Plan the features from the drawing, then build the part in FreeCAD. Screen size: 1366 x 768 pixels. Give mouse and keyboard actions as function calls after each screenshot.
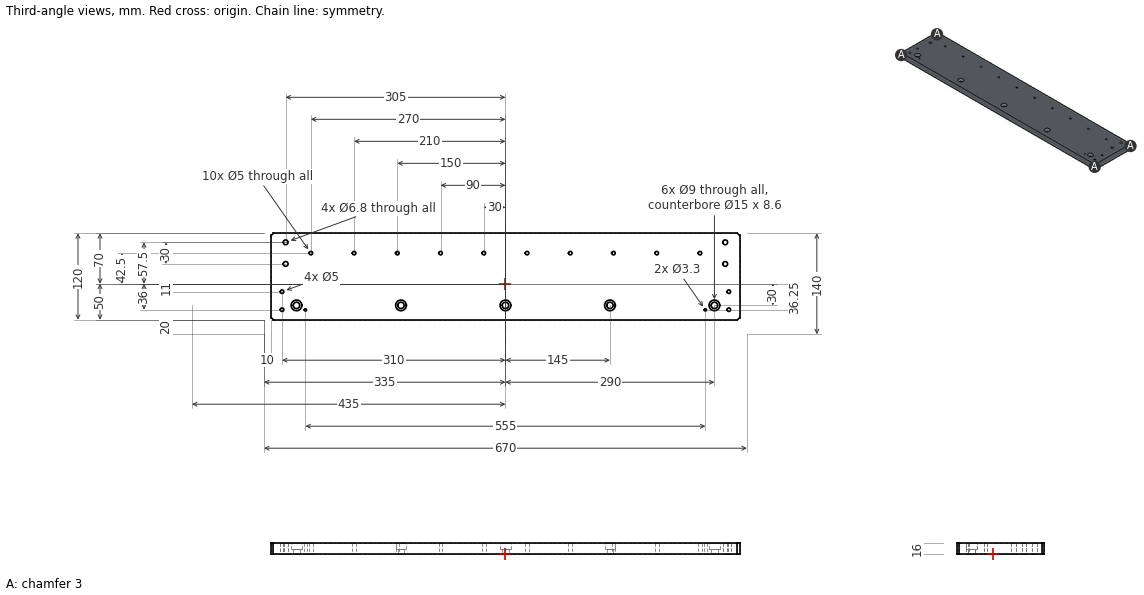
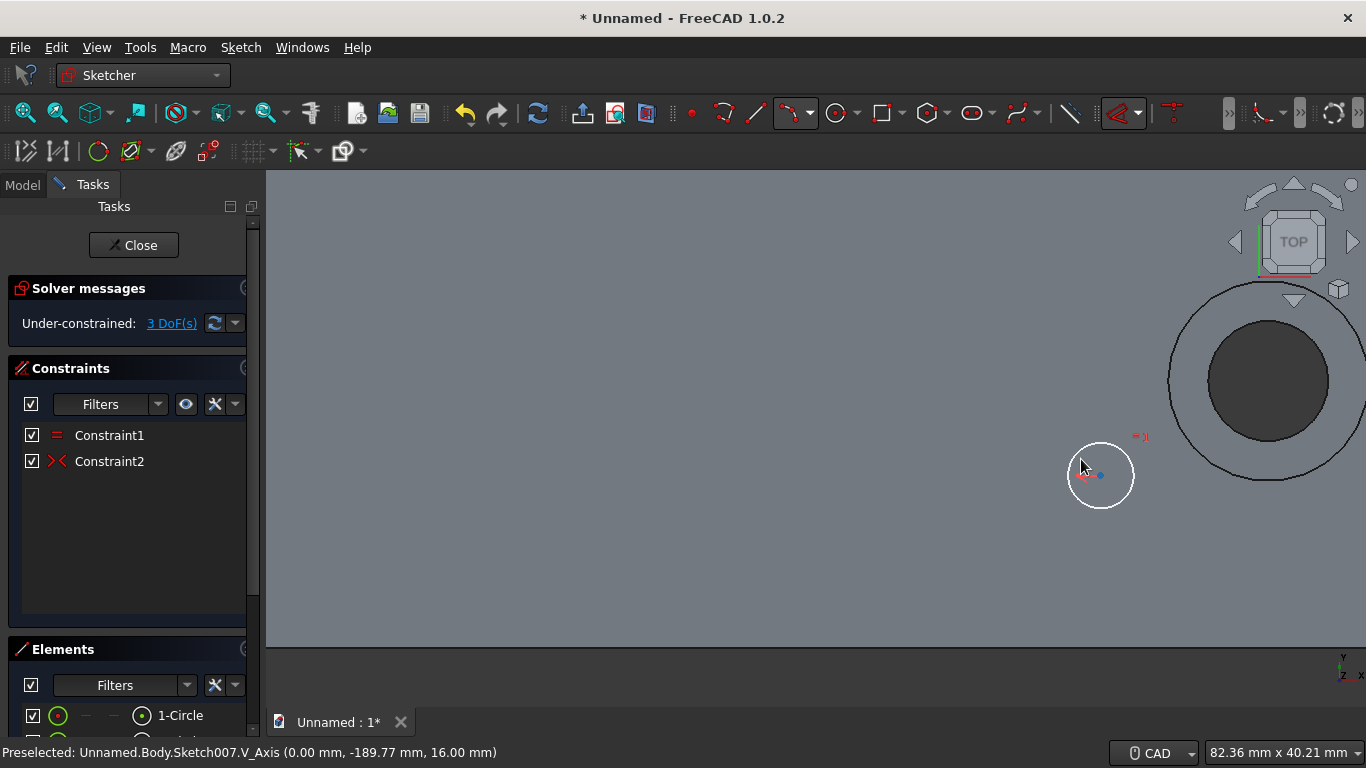
click(1078, 453)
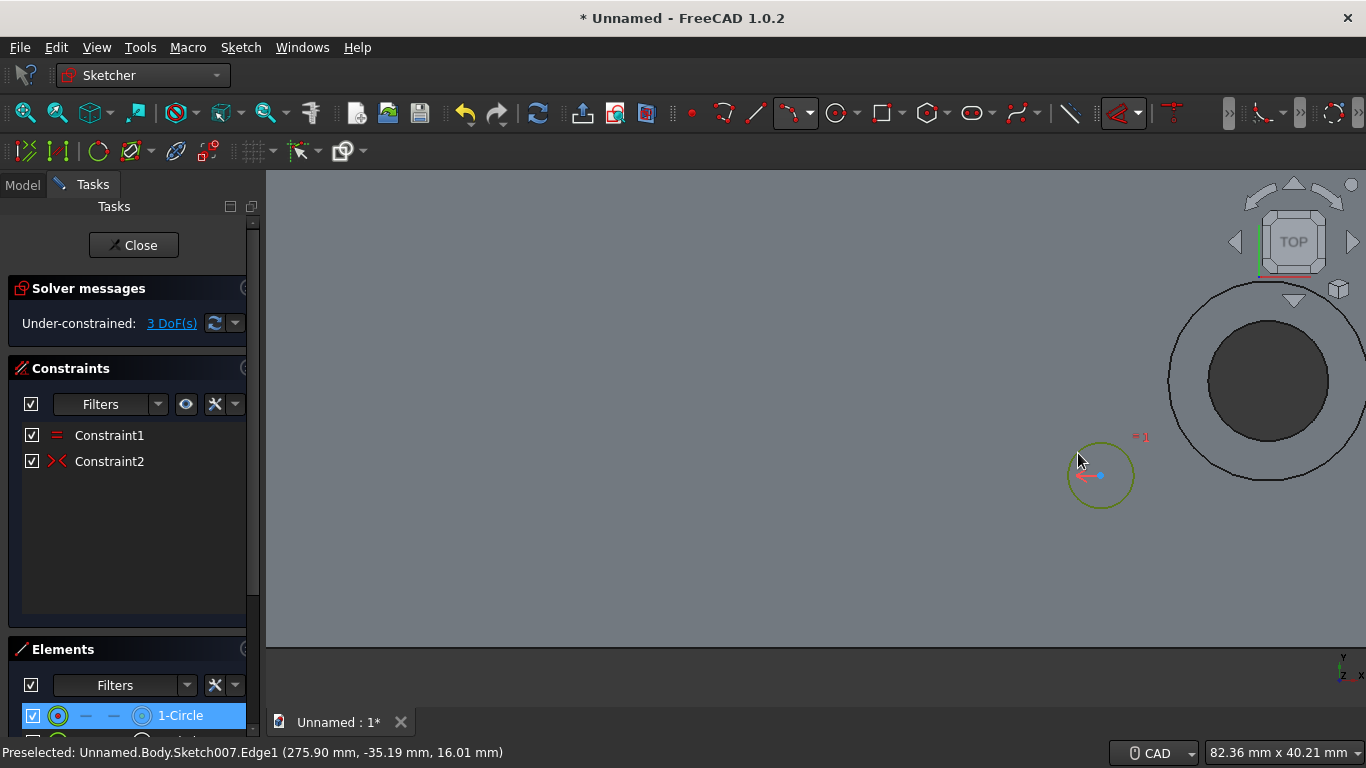
click(1140, 114)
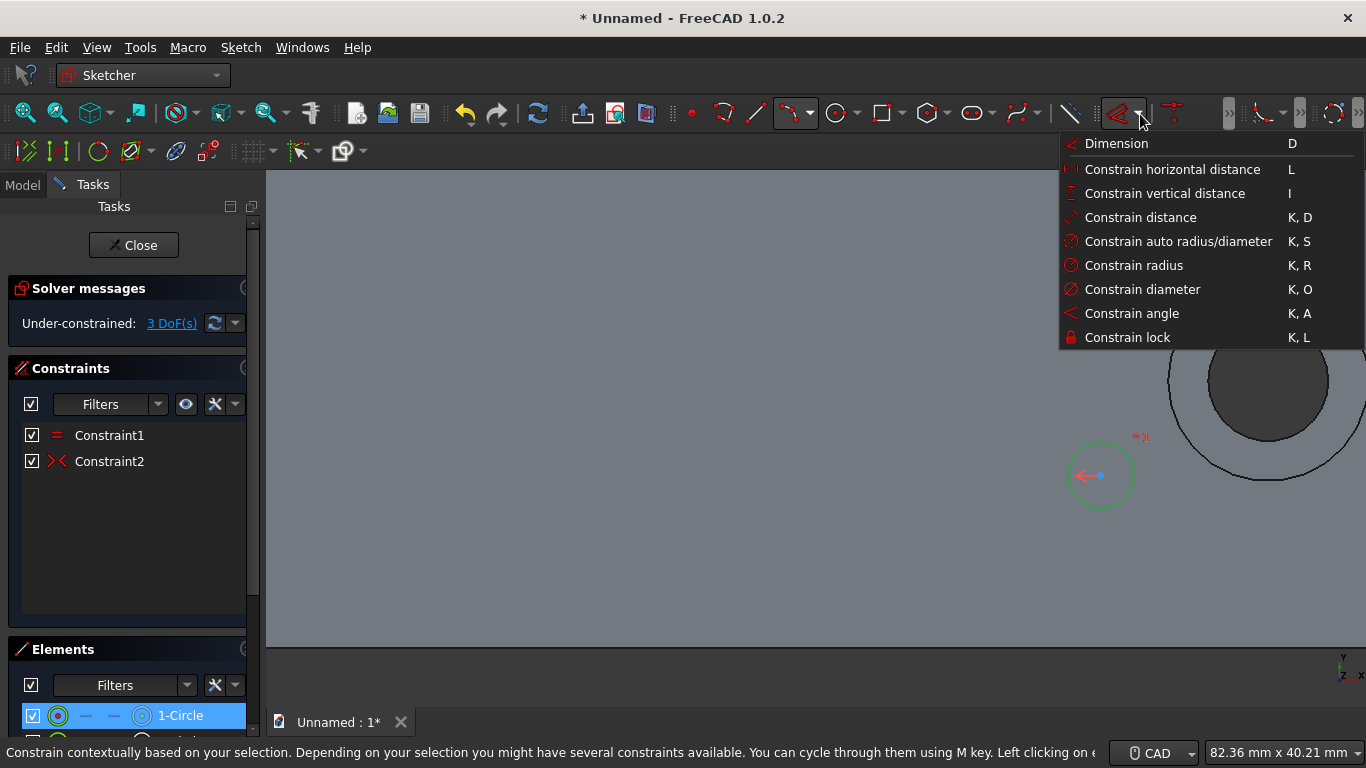
click(1212, 289)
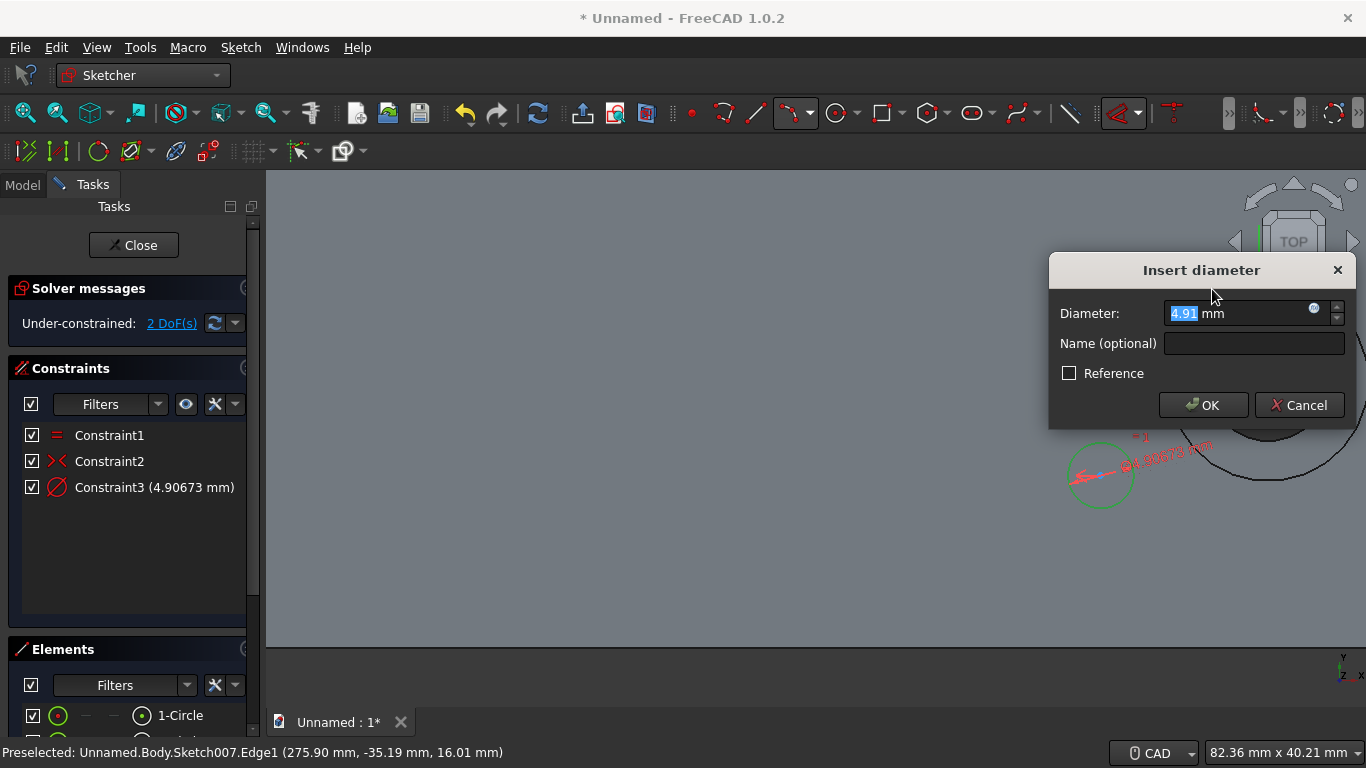
text(3.3)
key(Return)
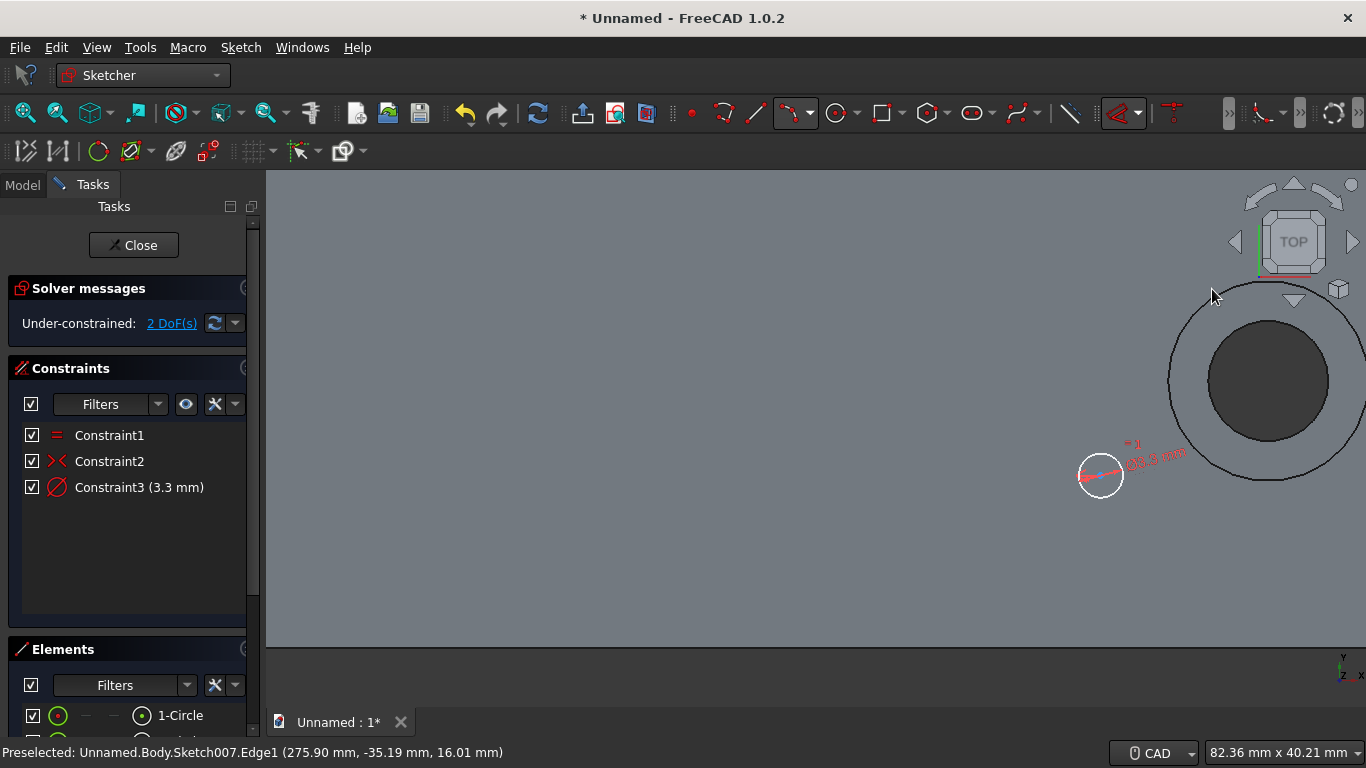
scroll(1082, 459, down, 12)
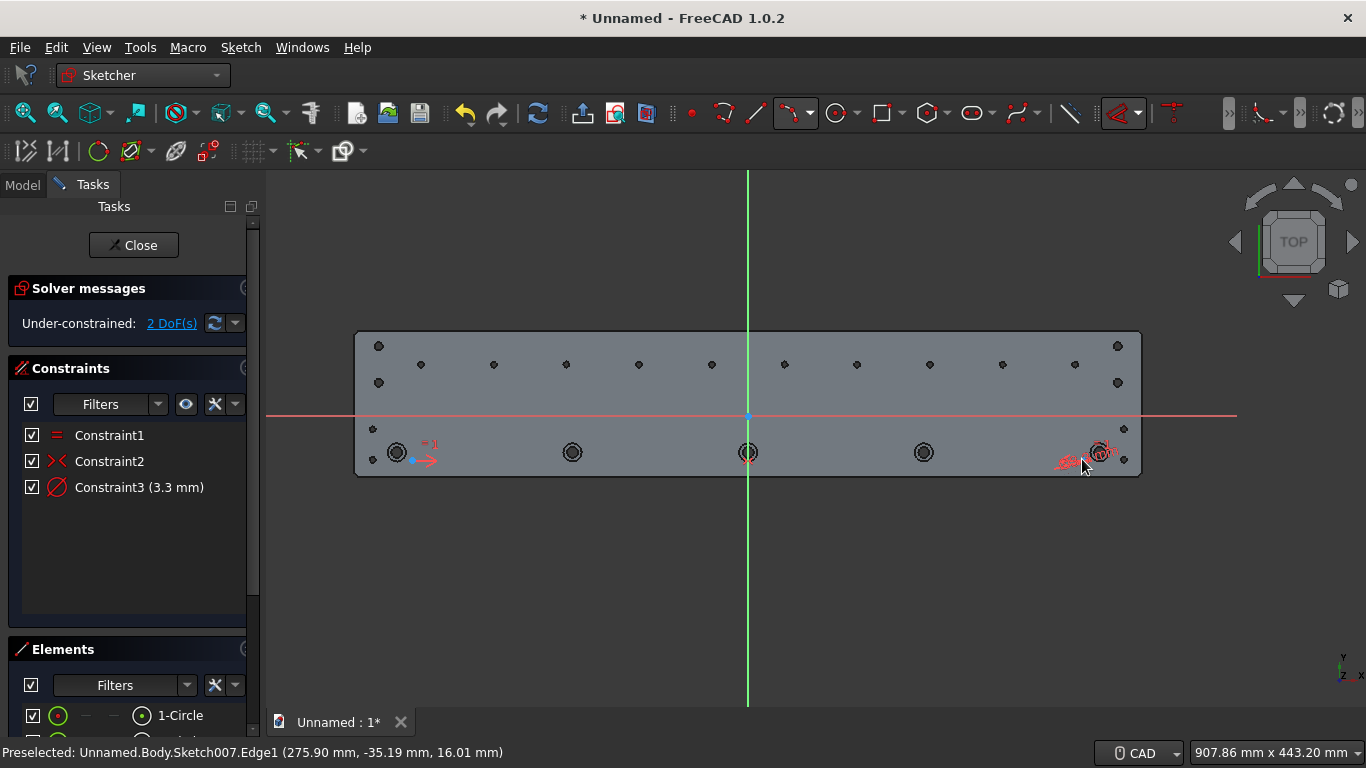
click(1084, 461)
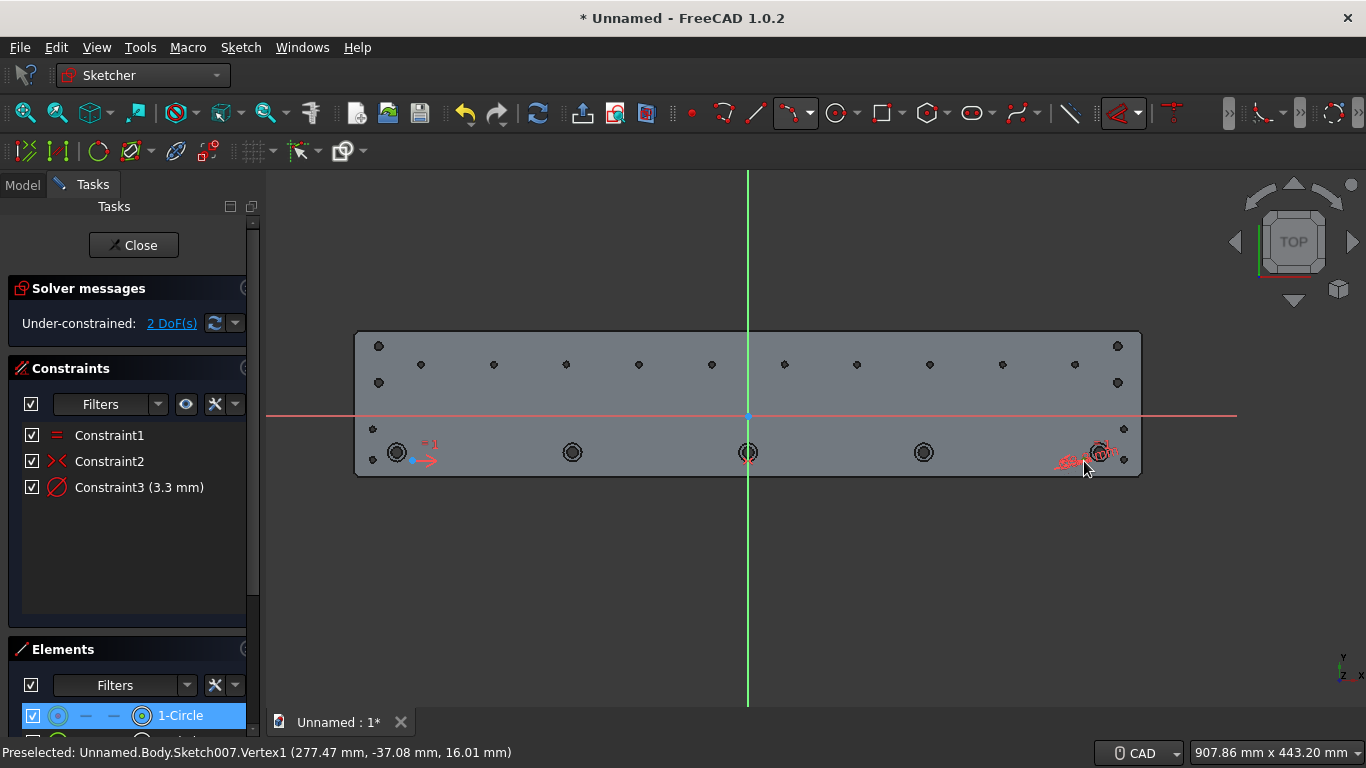
click(412, 461)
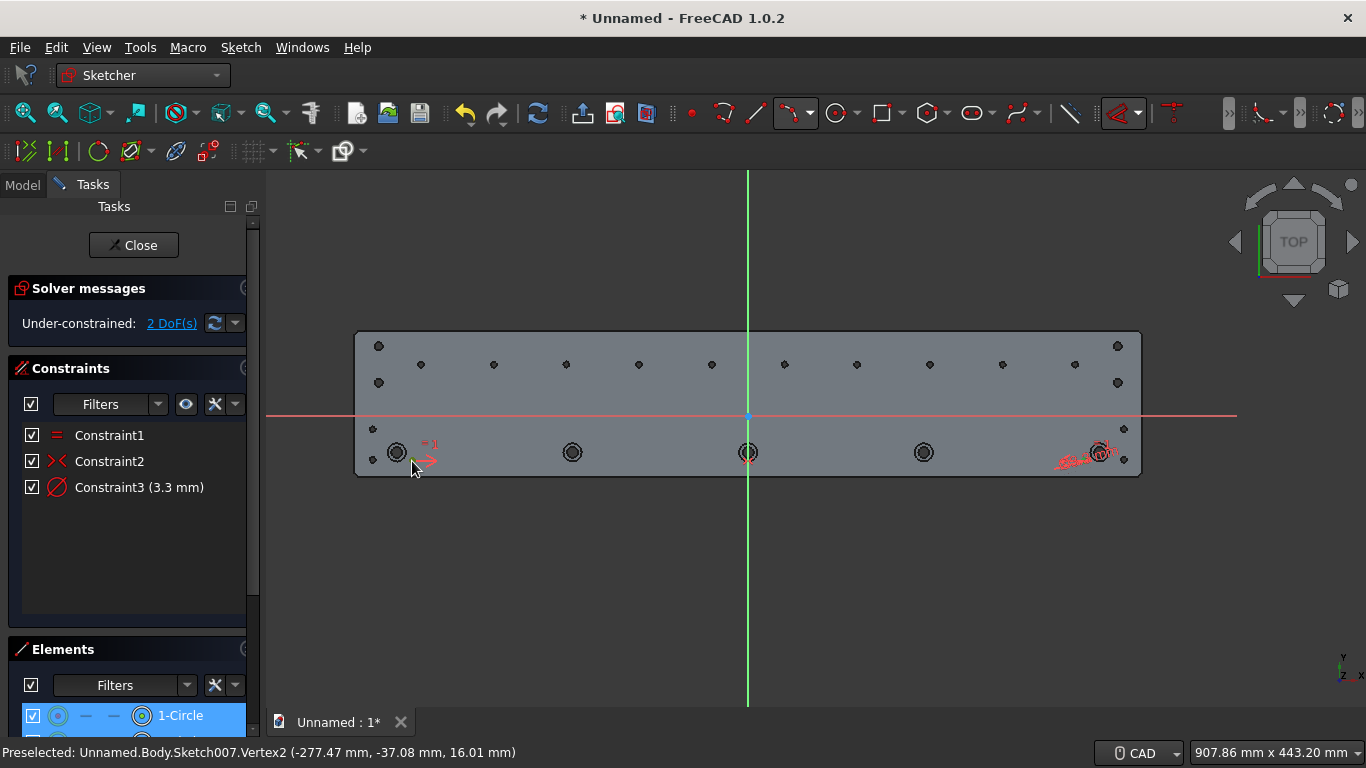
click(1140, 114)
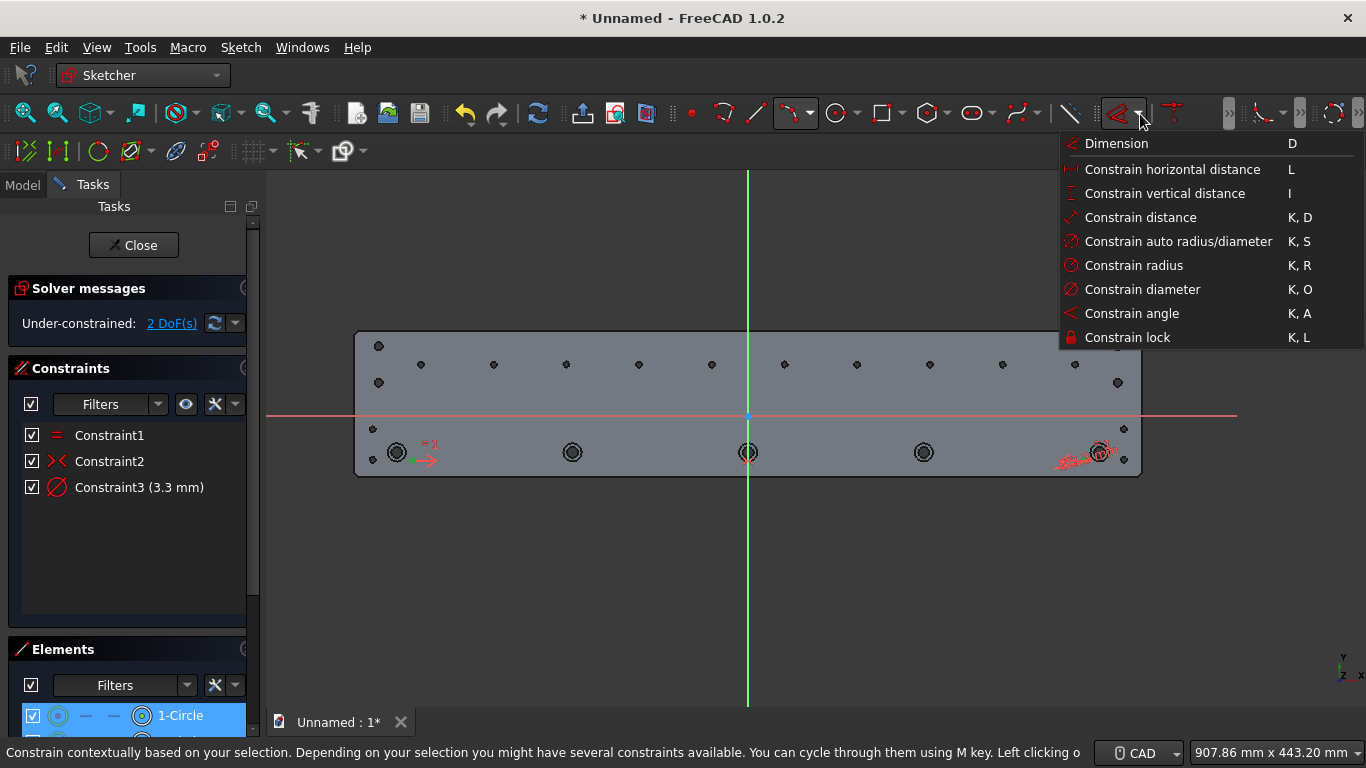
click(1212, 169)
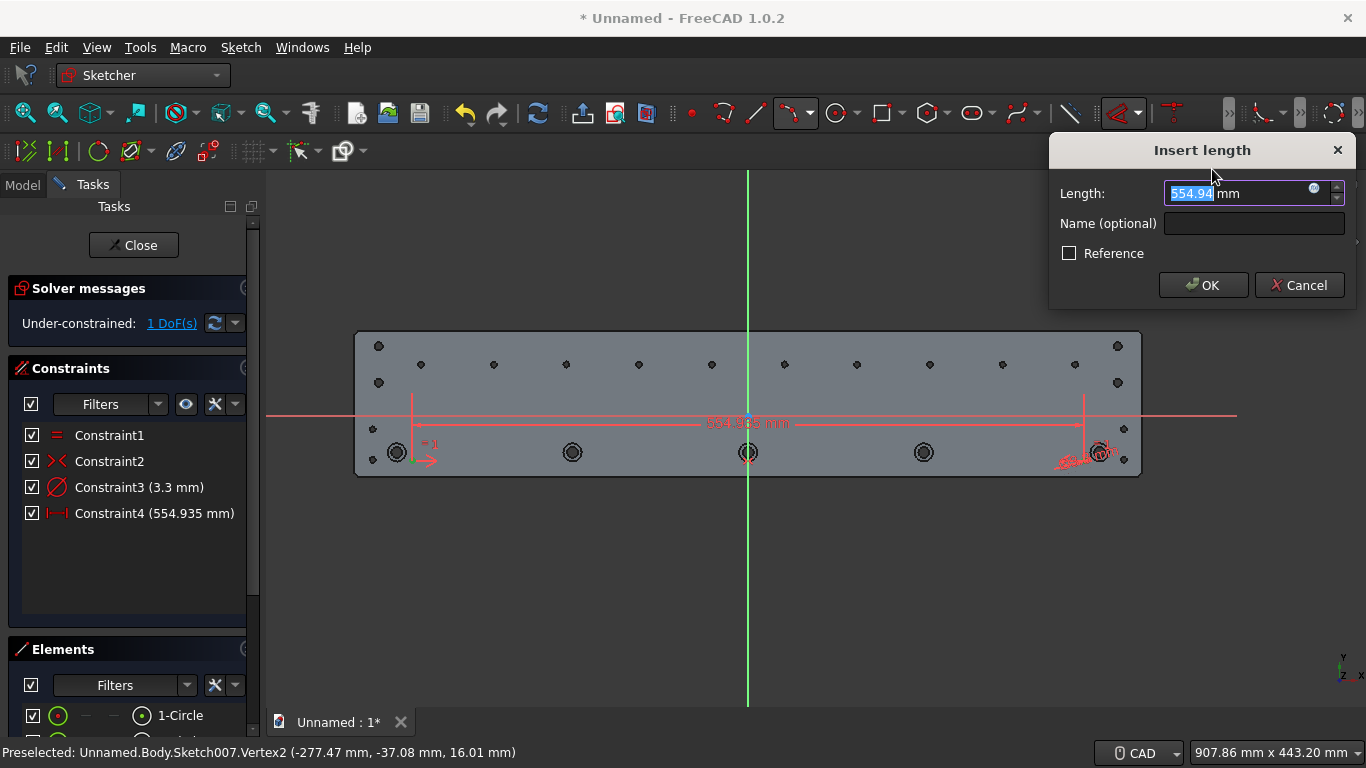
text(555)
key(Return)